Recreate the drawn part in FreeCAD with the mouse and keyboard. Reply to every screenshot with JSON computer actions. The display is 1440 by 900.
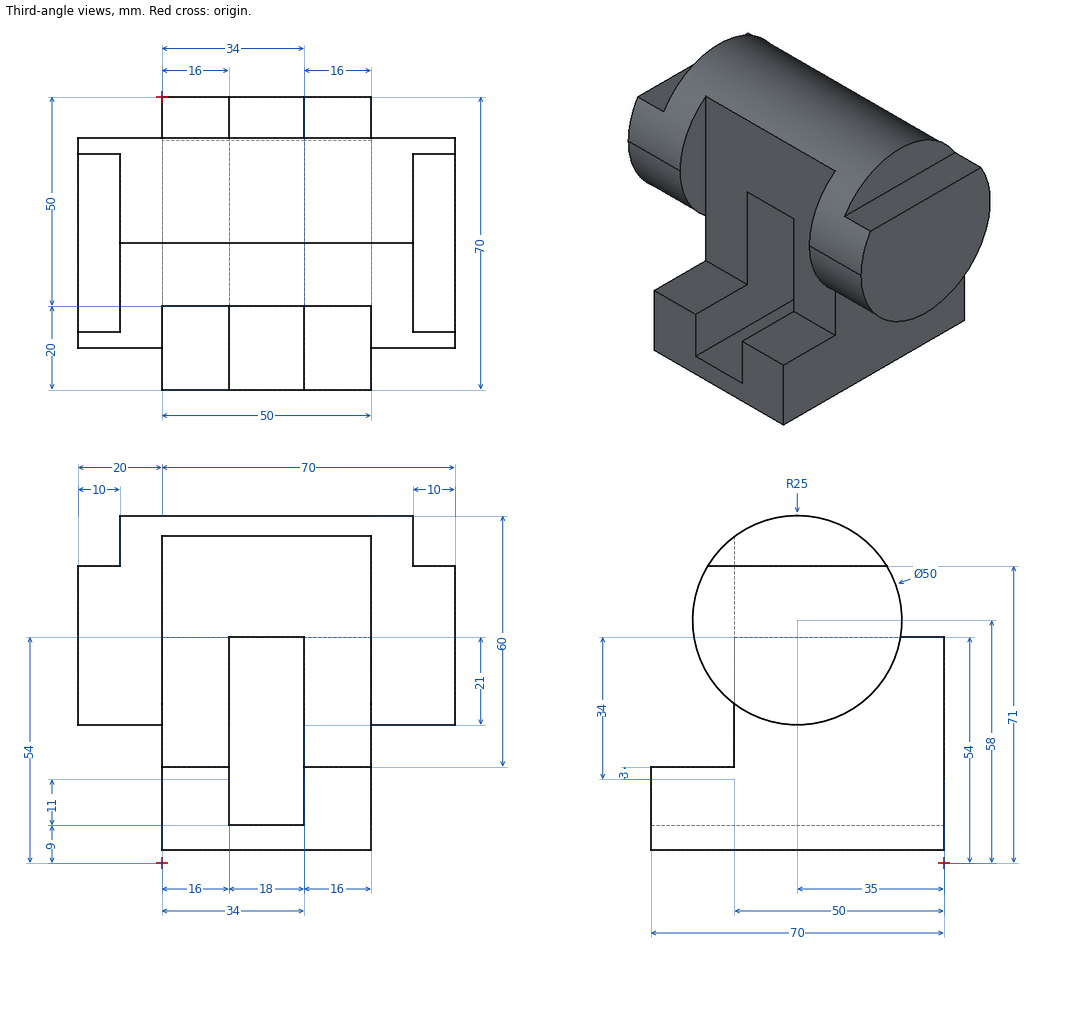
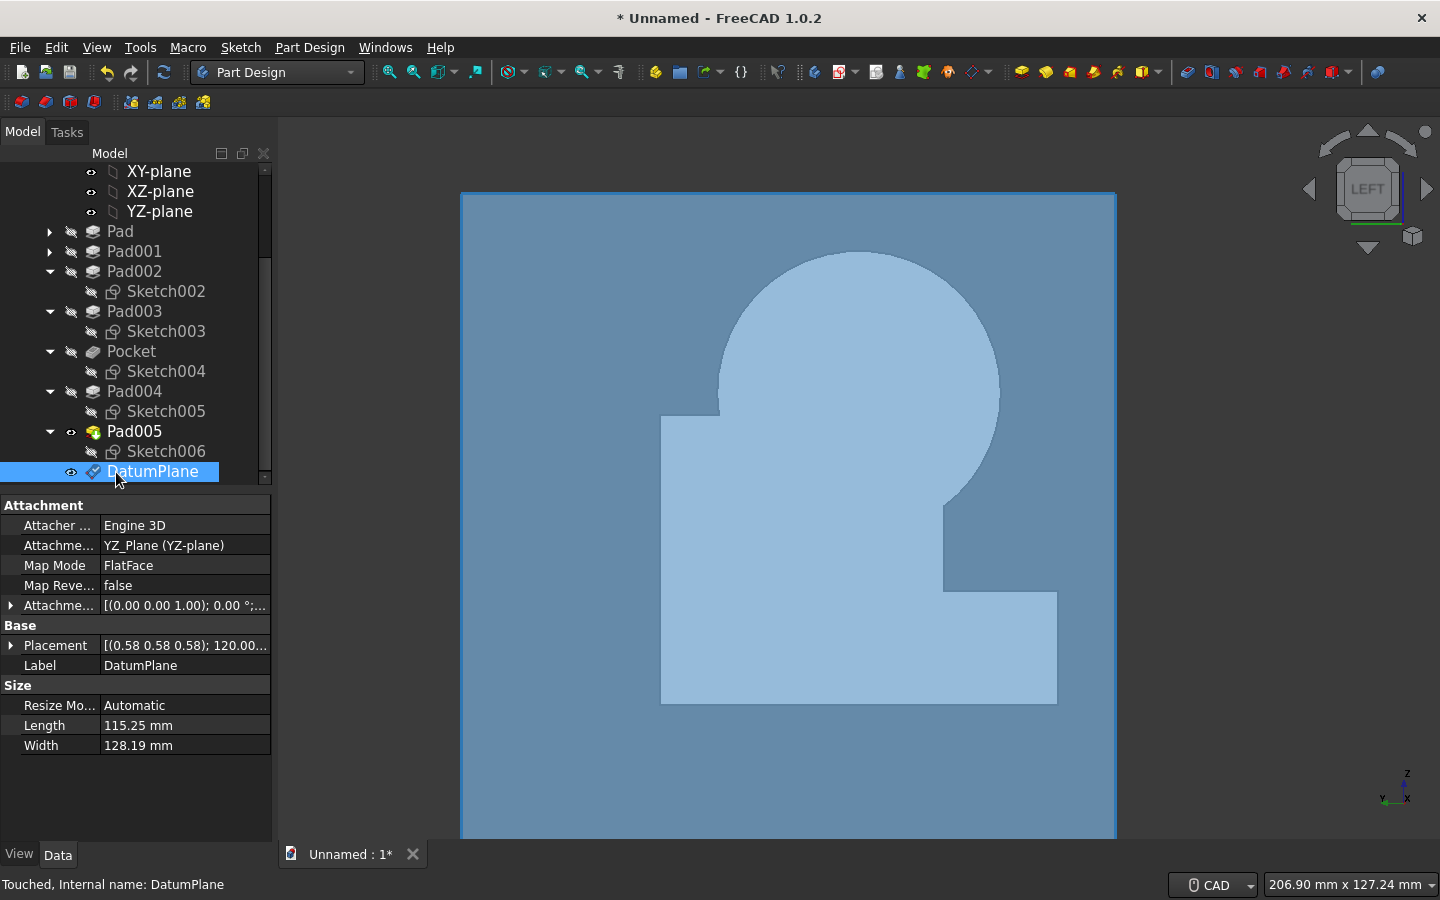
{"action": "left_click", "coordinate": [840, 72]}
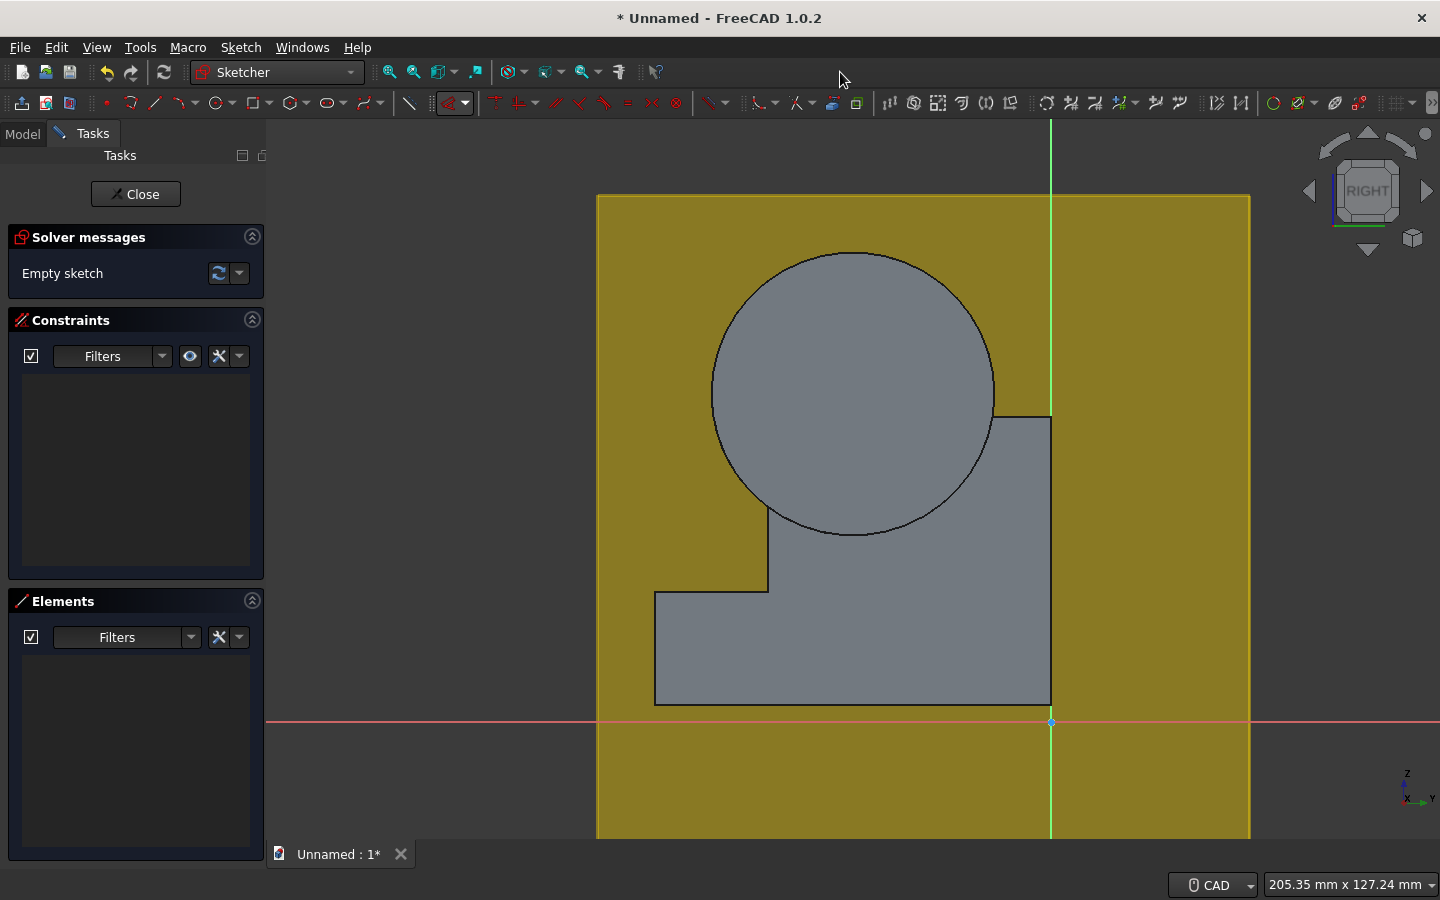
{"action": "left_click", "coordinate": [70, 104]}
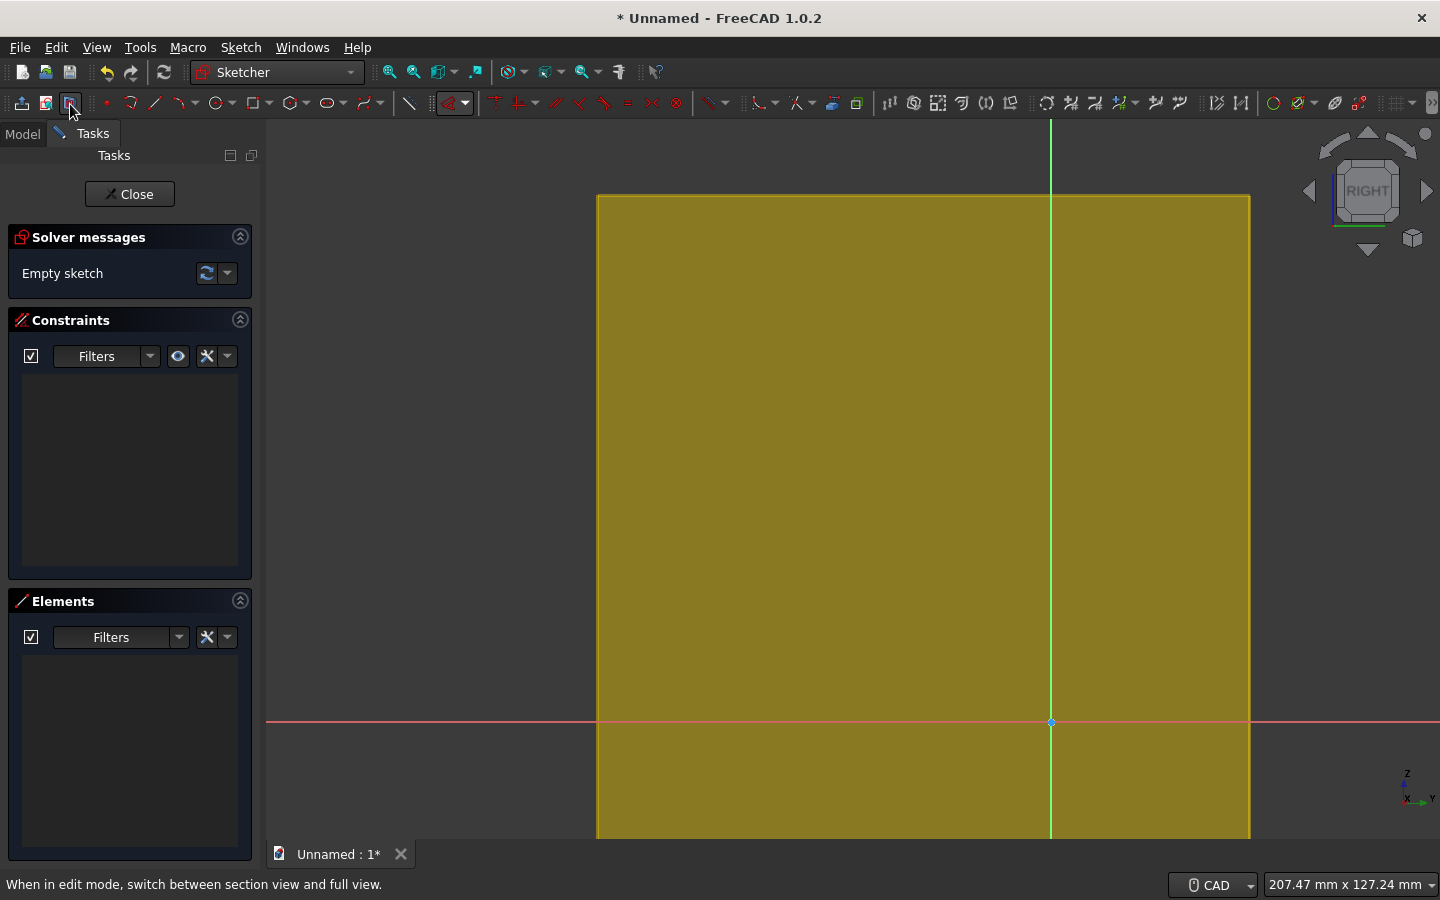
{"action": "left_click", "coordinate": [216, 104]}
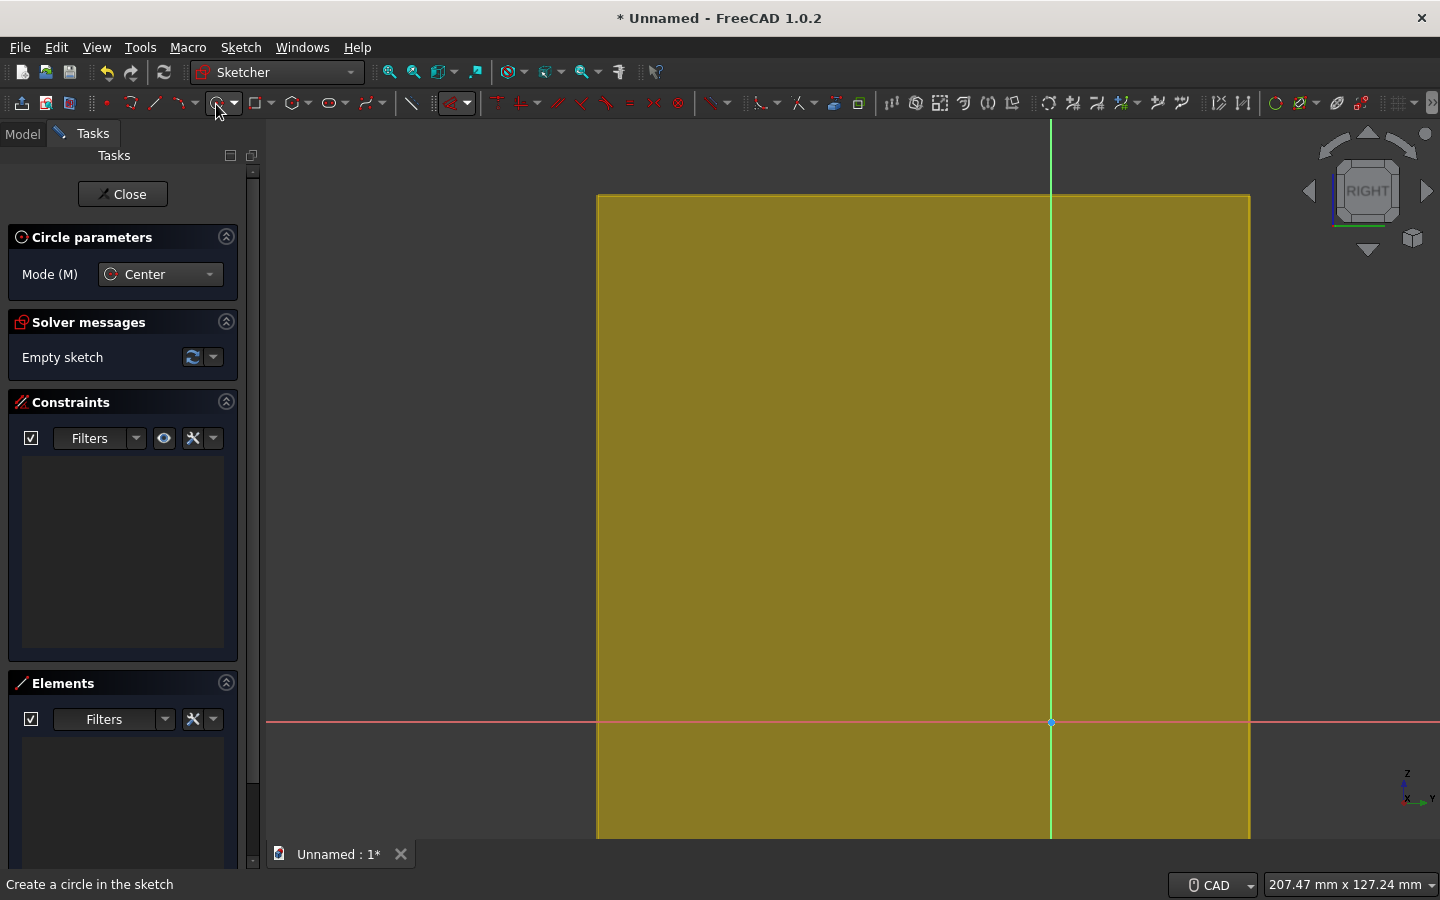
{"action": "left_click", "coordinate": [853, 394]}
{"action": "mouse_move", "coordinate": [953, 294]}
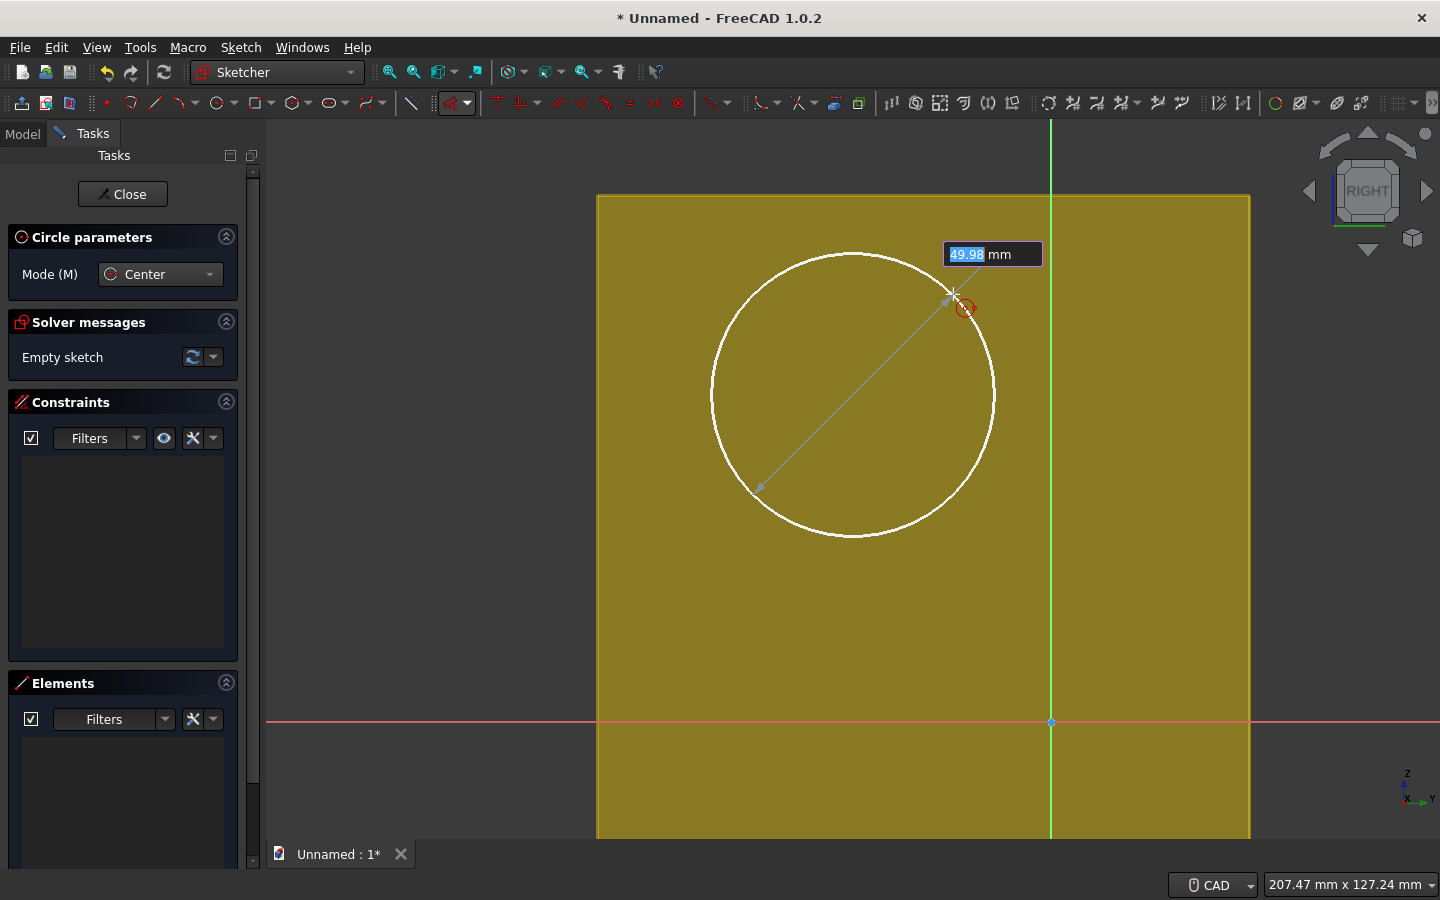
{"action": "type", "text": "50"}
{"action": "key", "text": "Return"}
{"action": "key", "text": "Escape"}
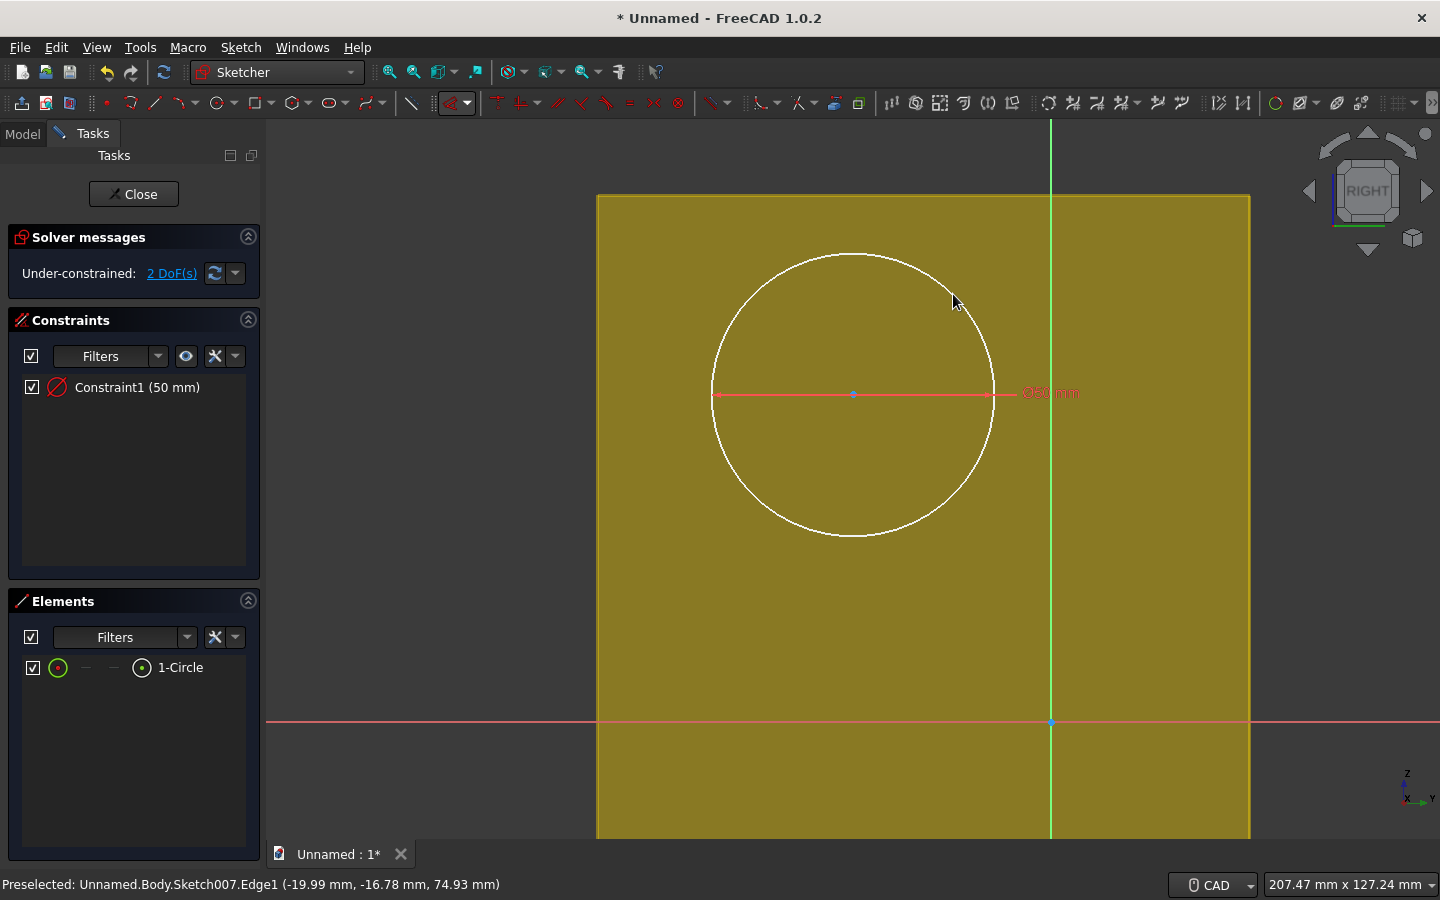
{"action": "left_click", "coordinate": [853, 395]}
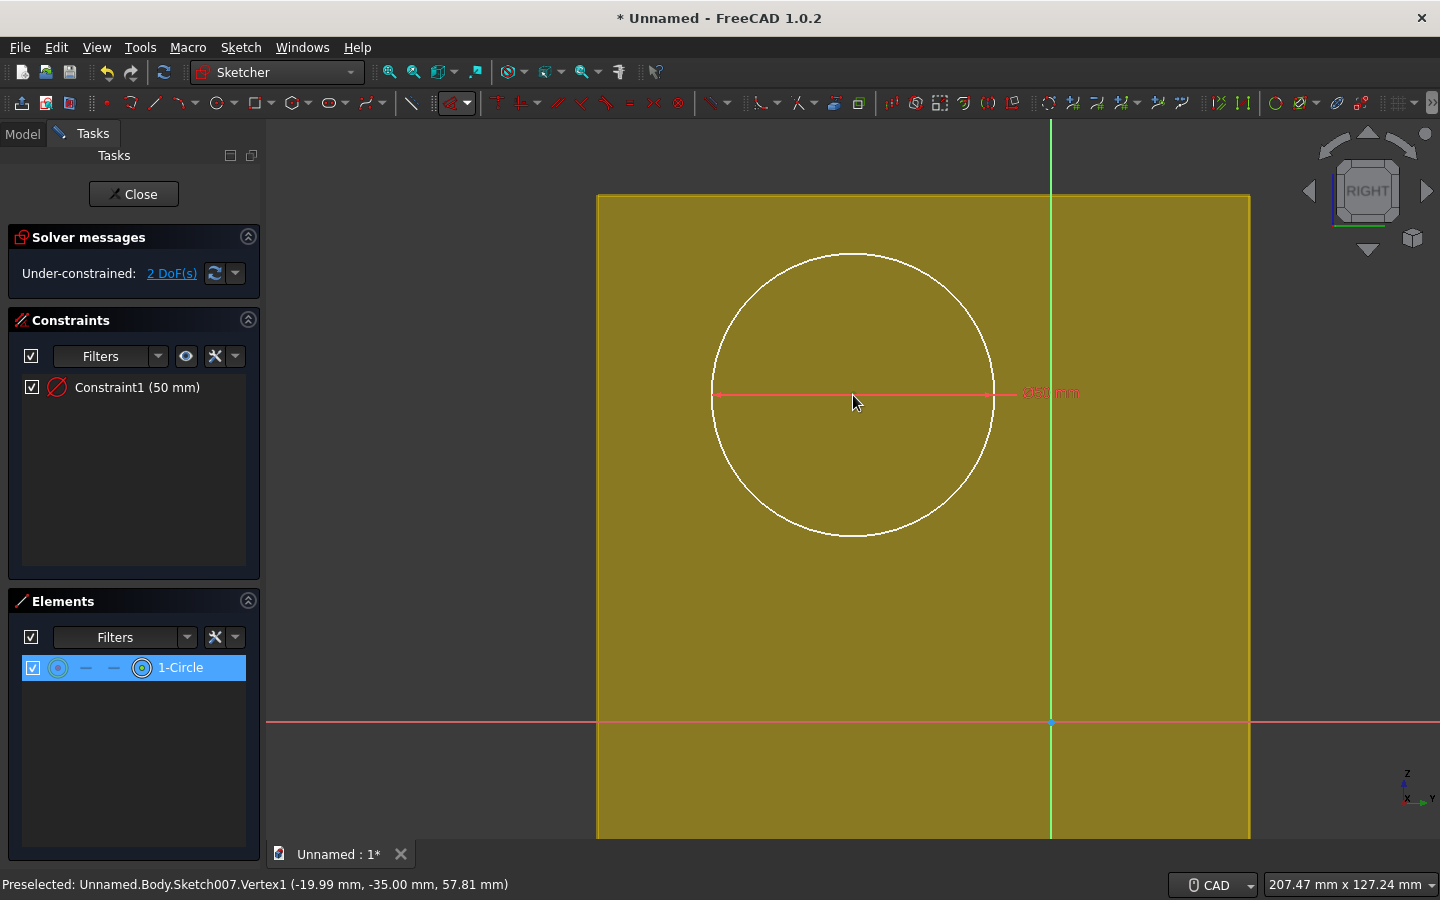
{"action": "left_click", "coordinate": [470, 104]}